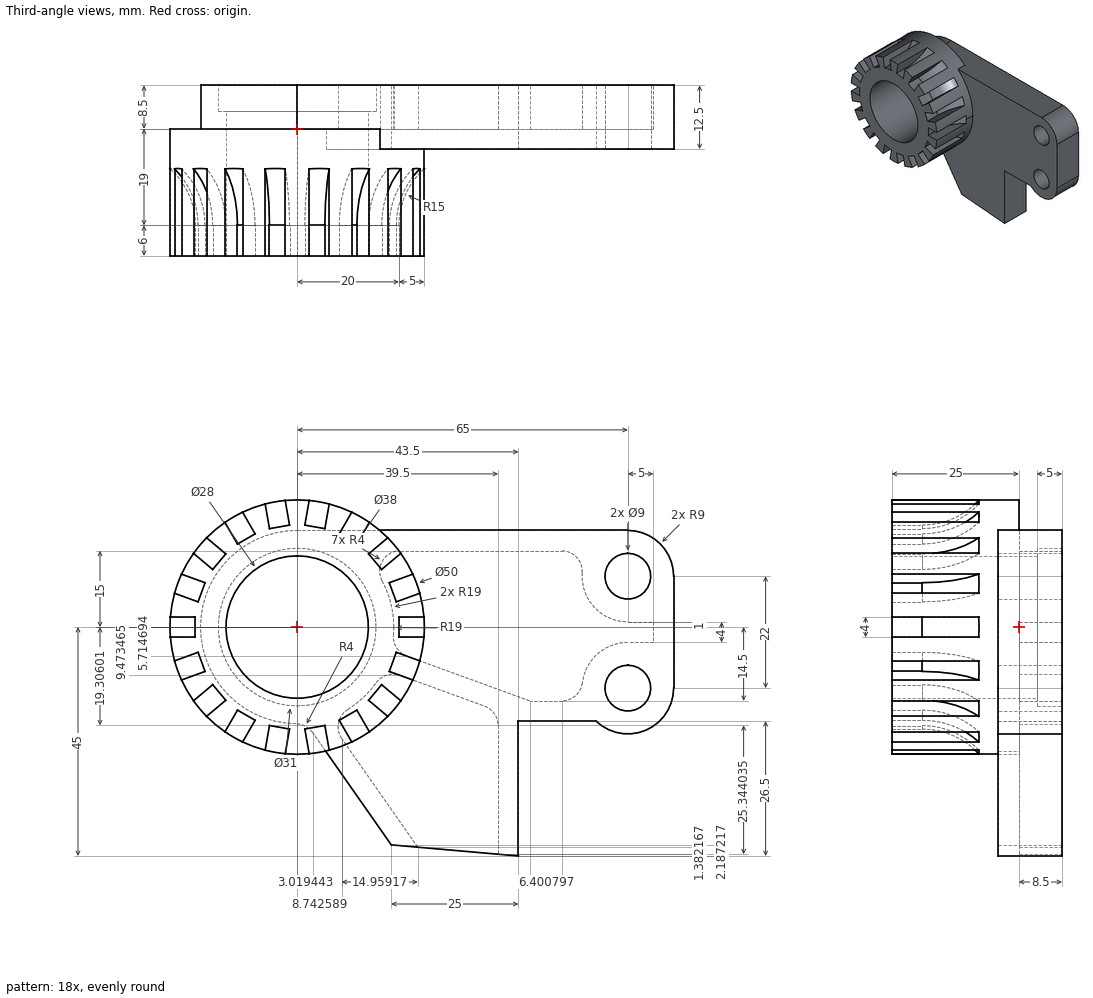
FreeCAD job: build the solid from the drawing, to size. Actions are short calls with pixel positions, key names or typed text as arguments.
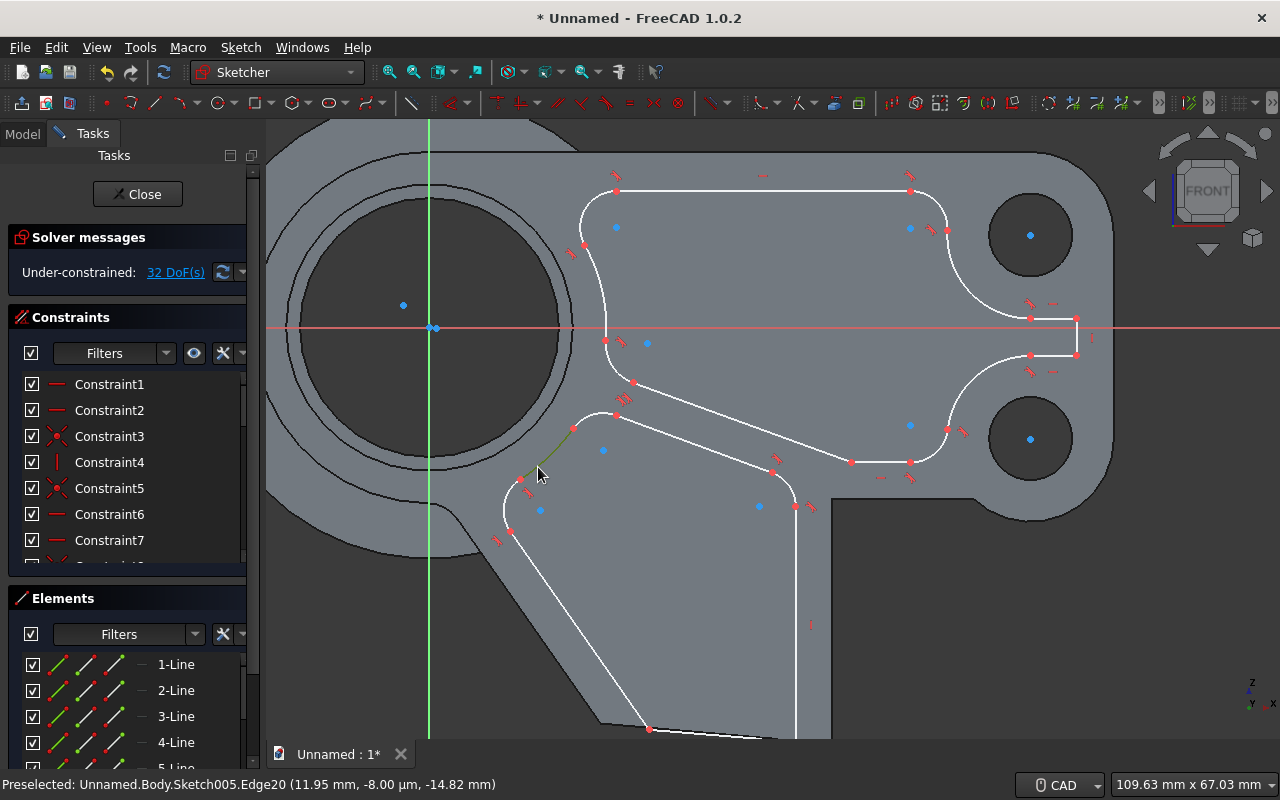
click(602, 413)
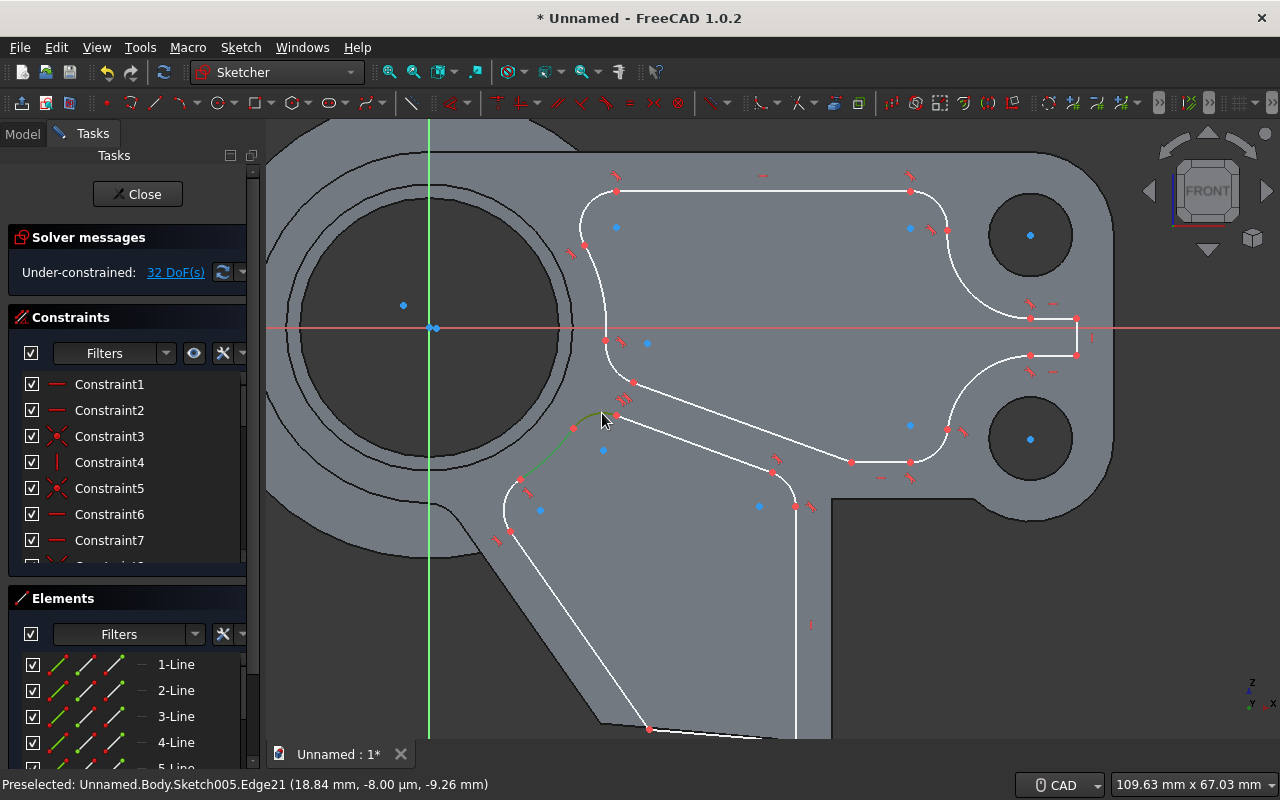
click(606, 104)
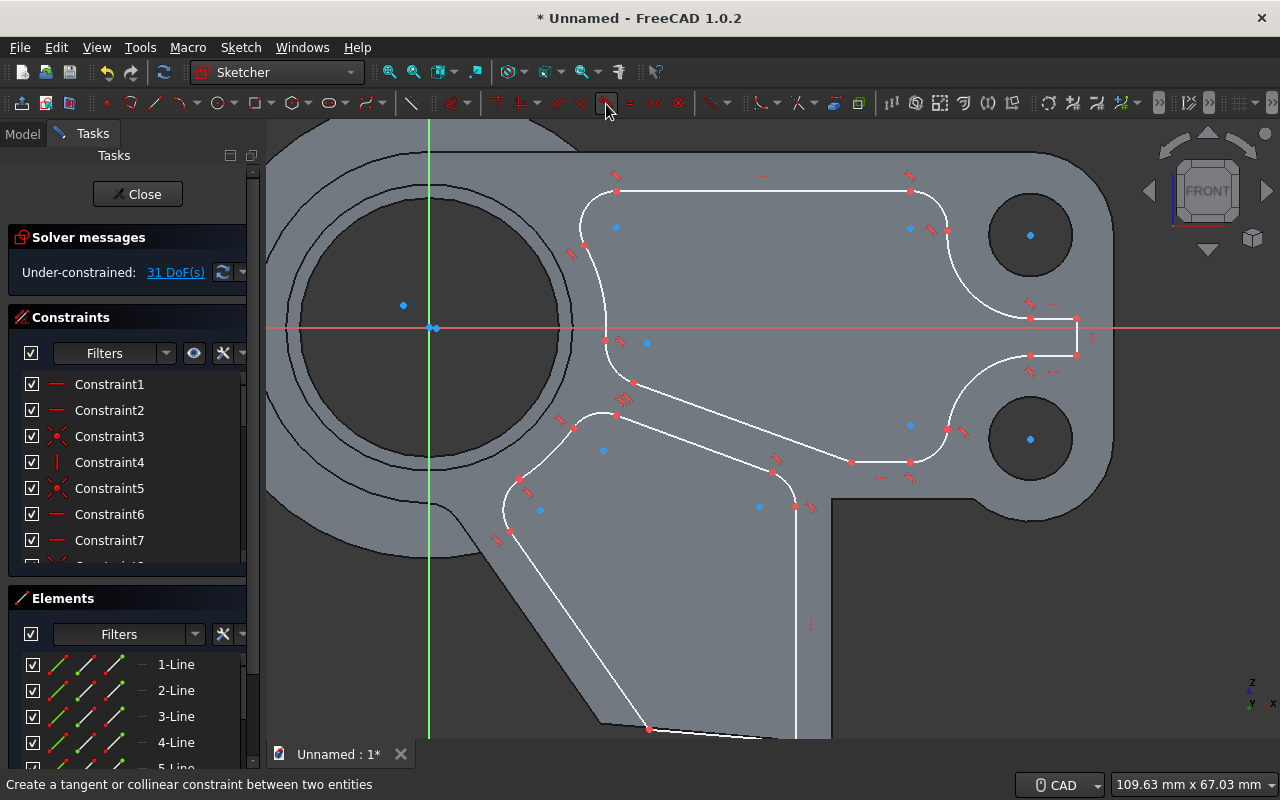
click(606, 311)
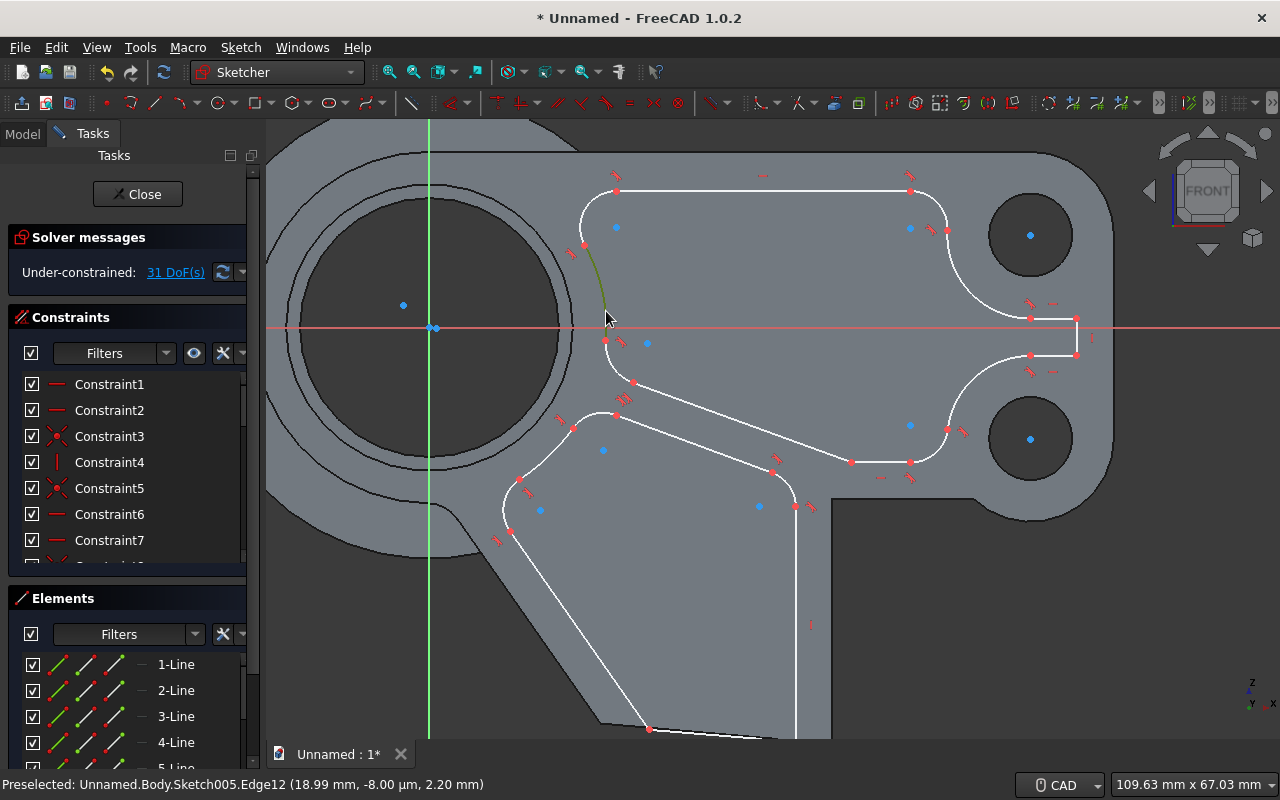
click(538, 466)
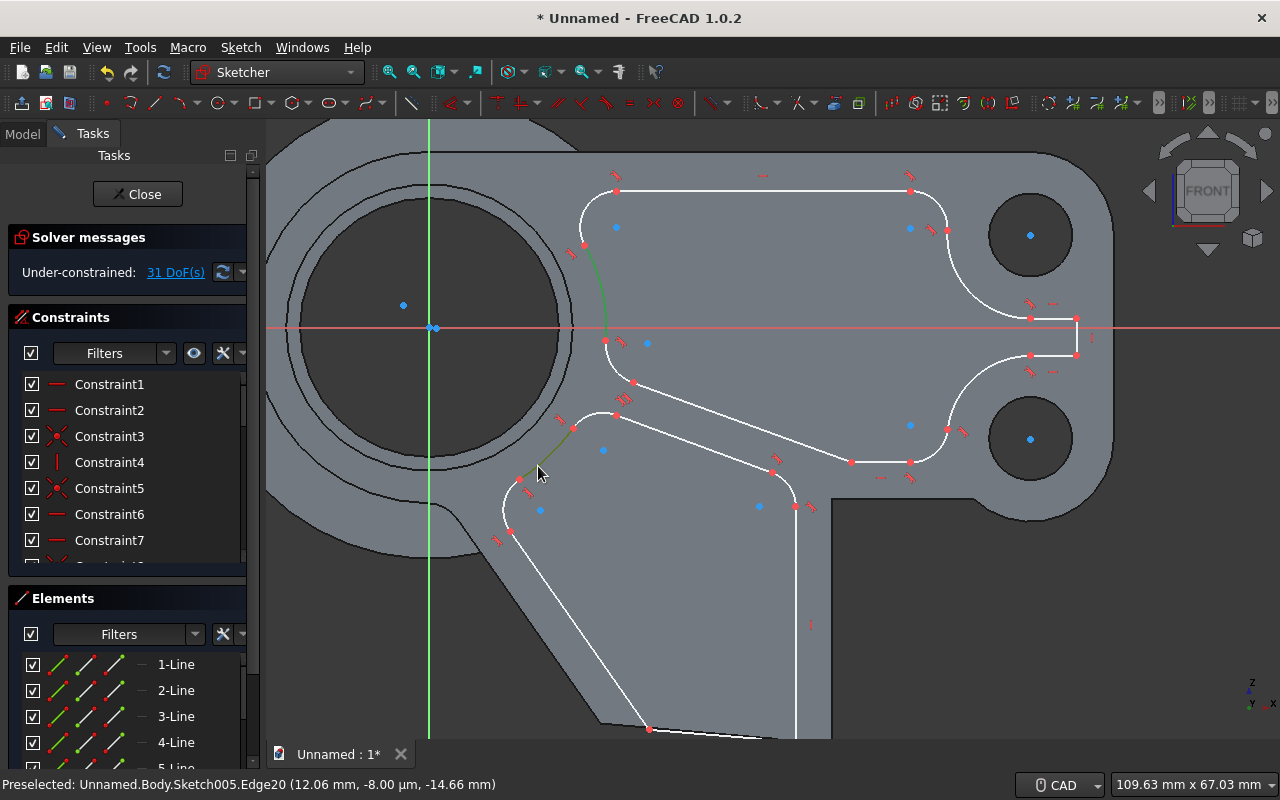
click(498, 104)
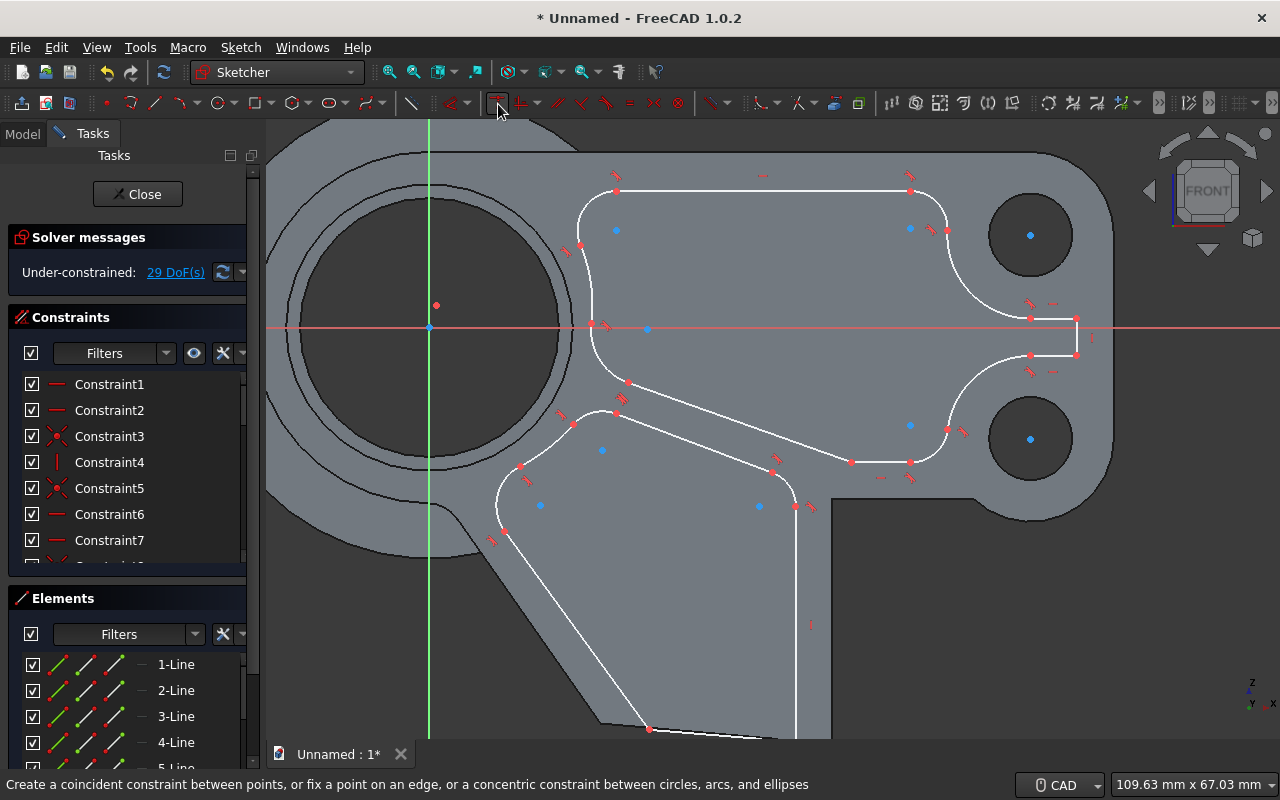
drag(419, 295, 446, 338)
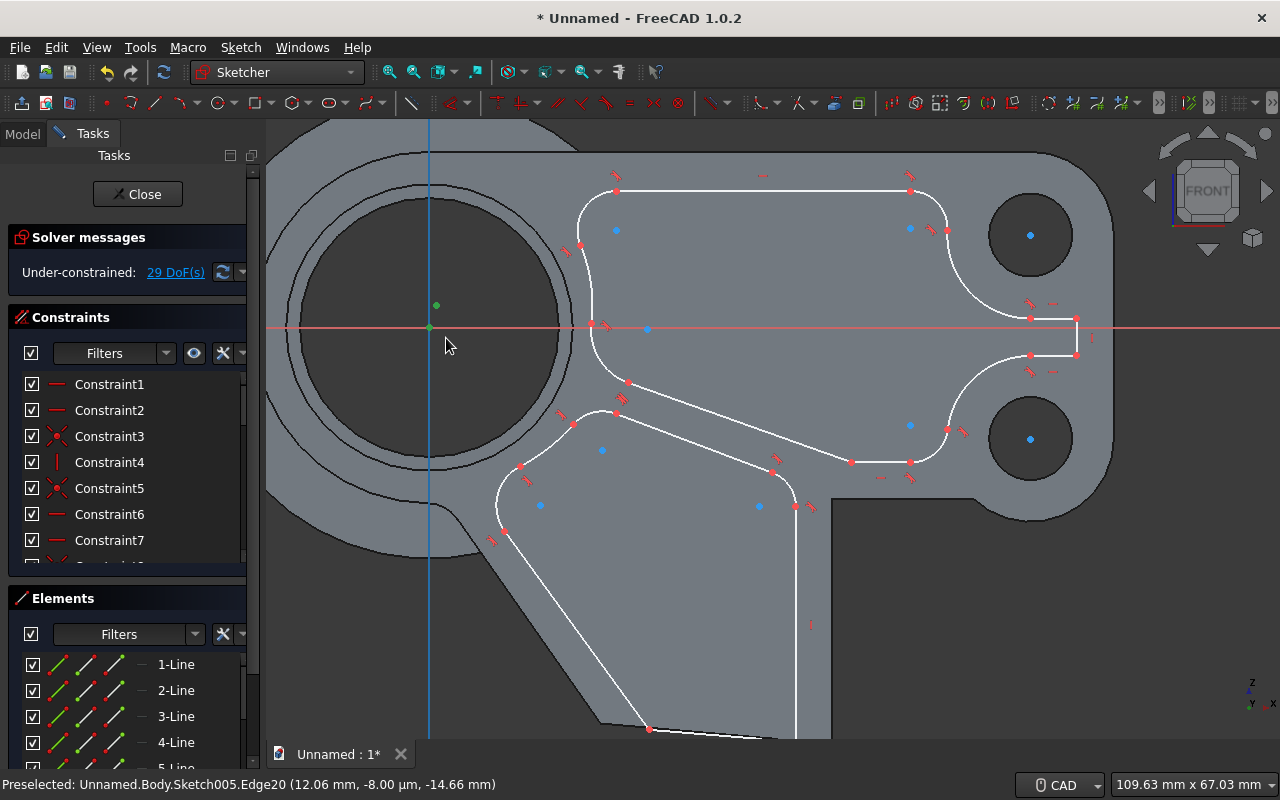
click(498, 104)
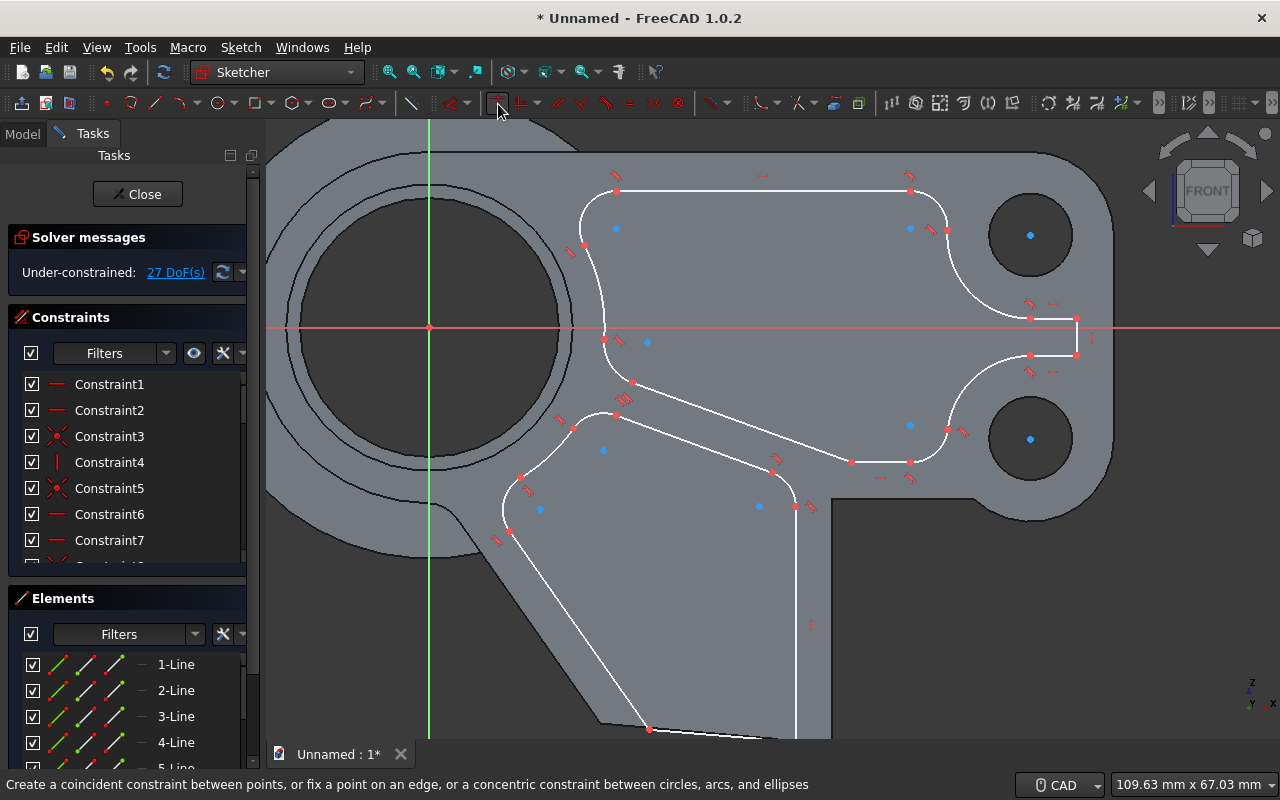
click(955, 270)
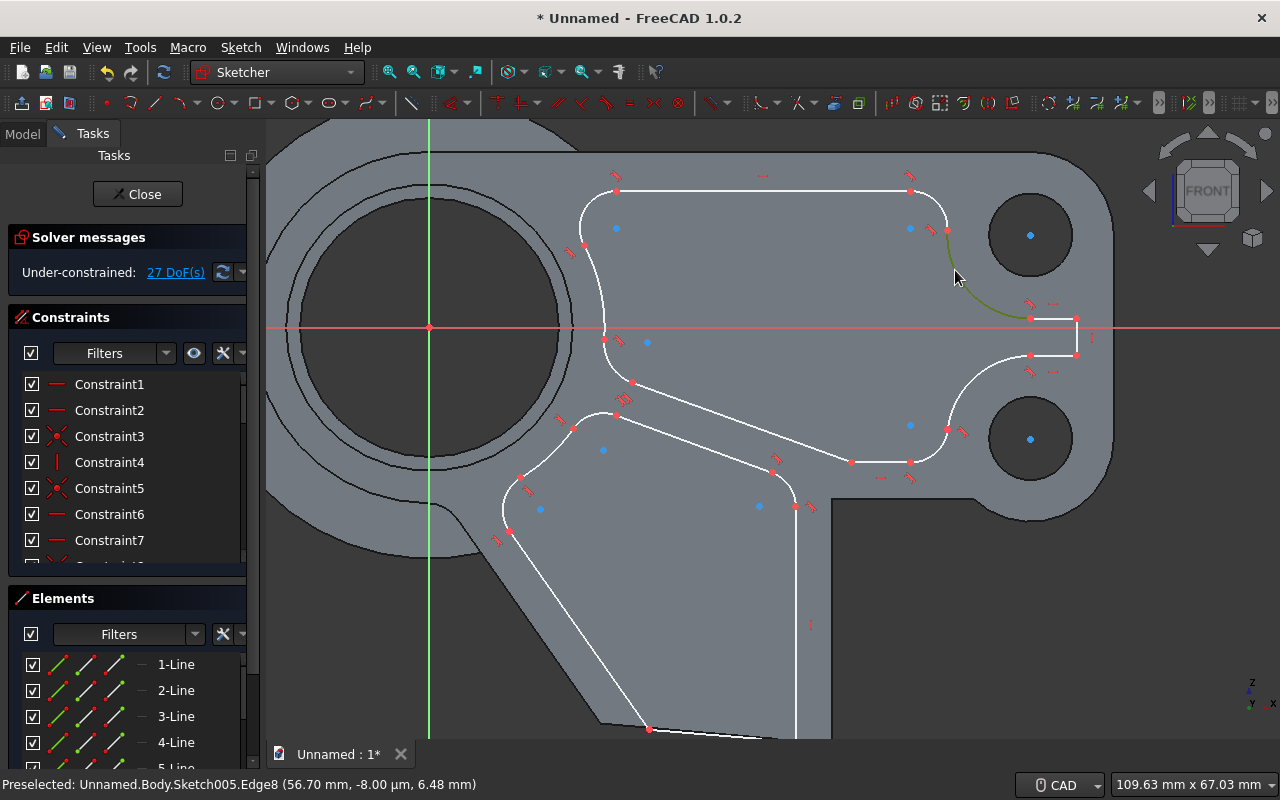
click(996, 364)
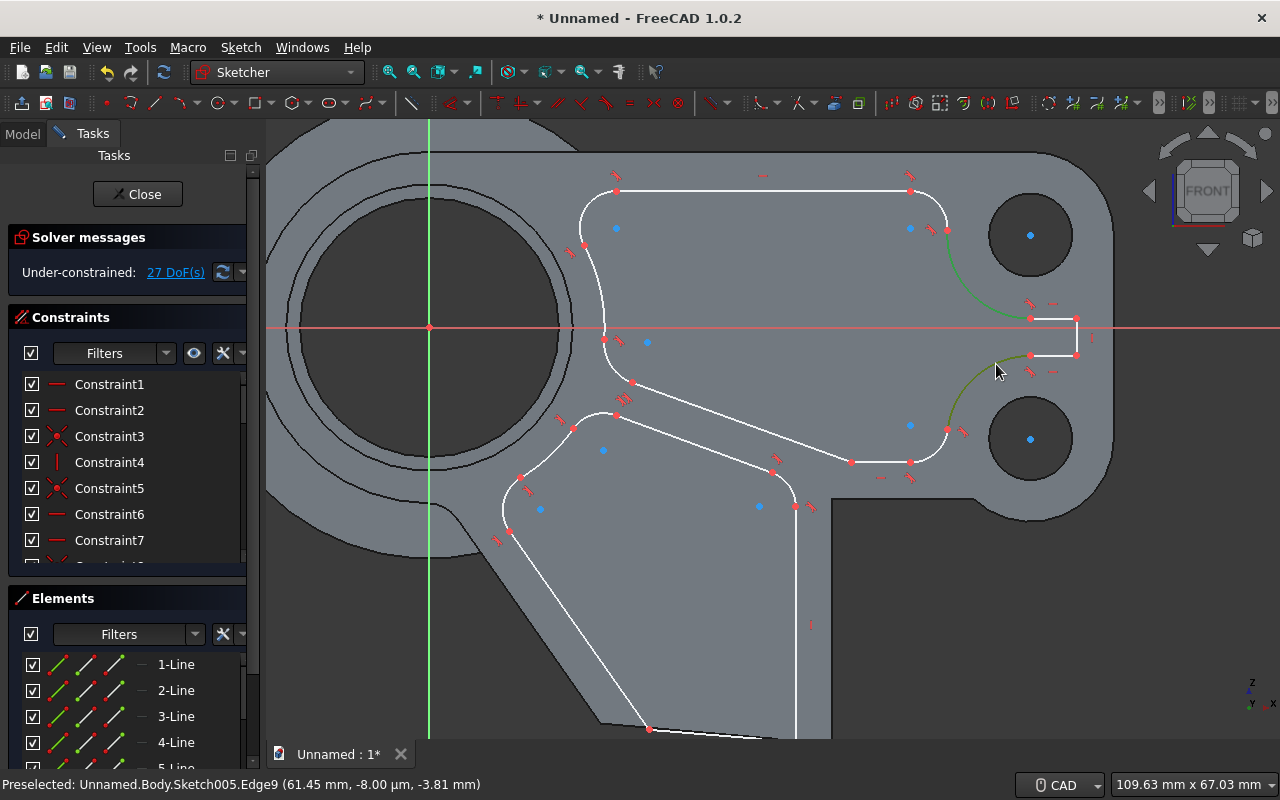
click(630, 104)